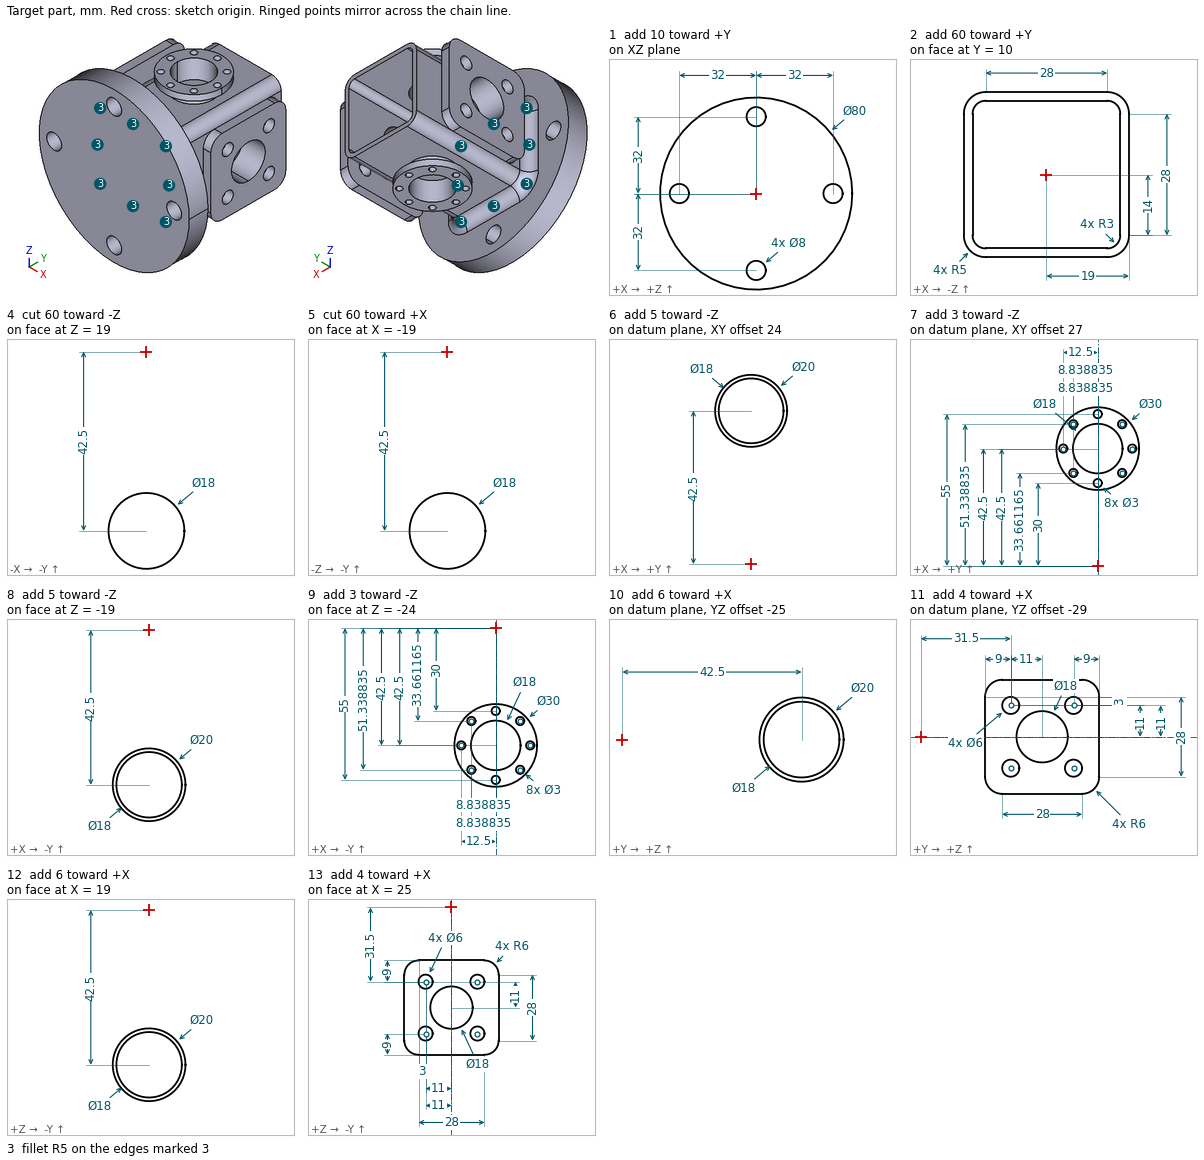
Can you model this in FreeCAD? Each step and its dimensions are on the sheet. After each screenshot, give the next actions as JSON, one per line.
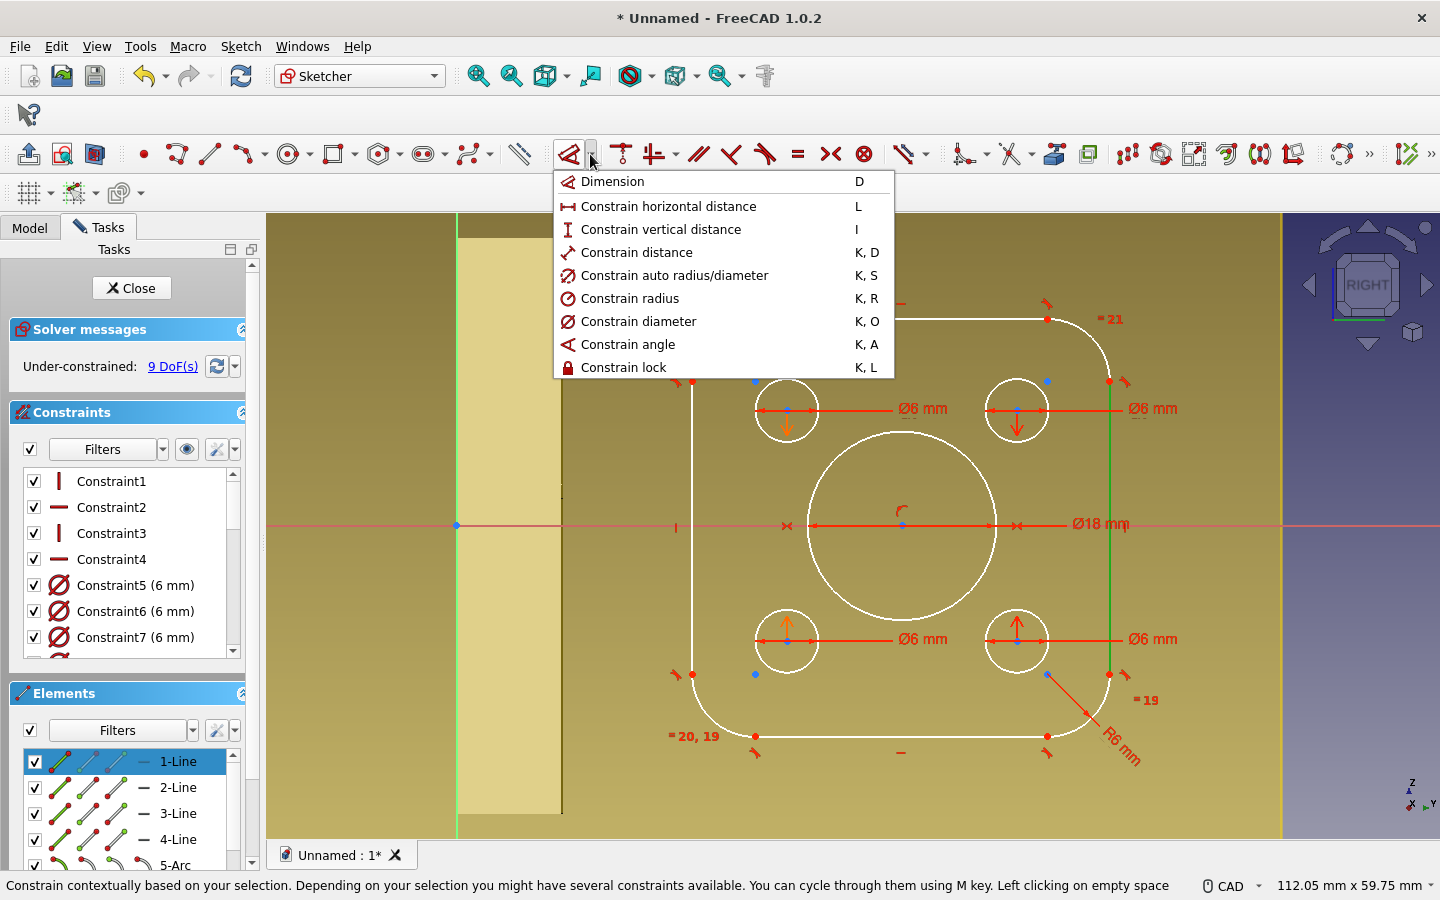
{"action": "left_click", "coordinate": [724, 230]}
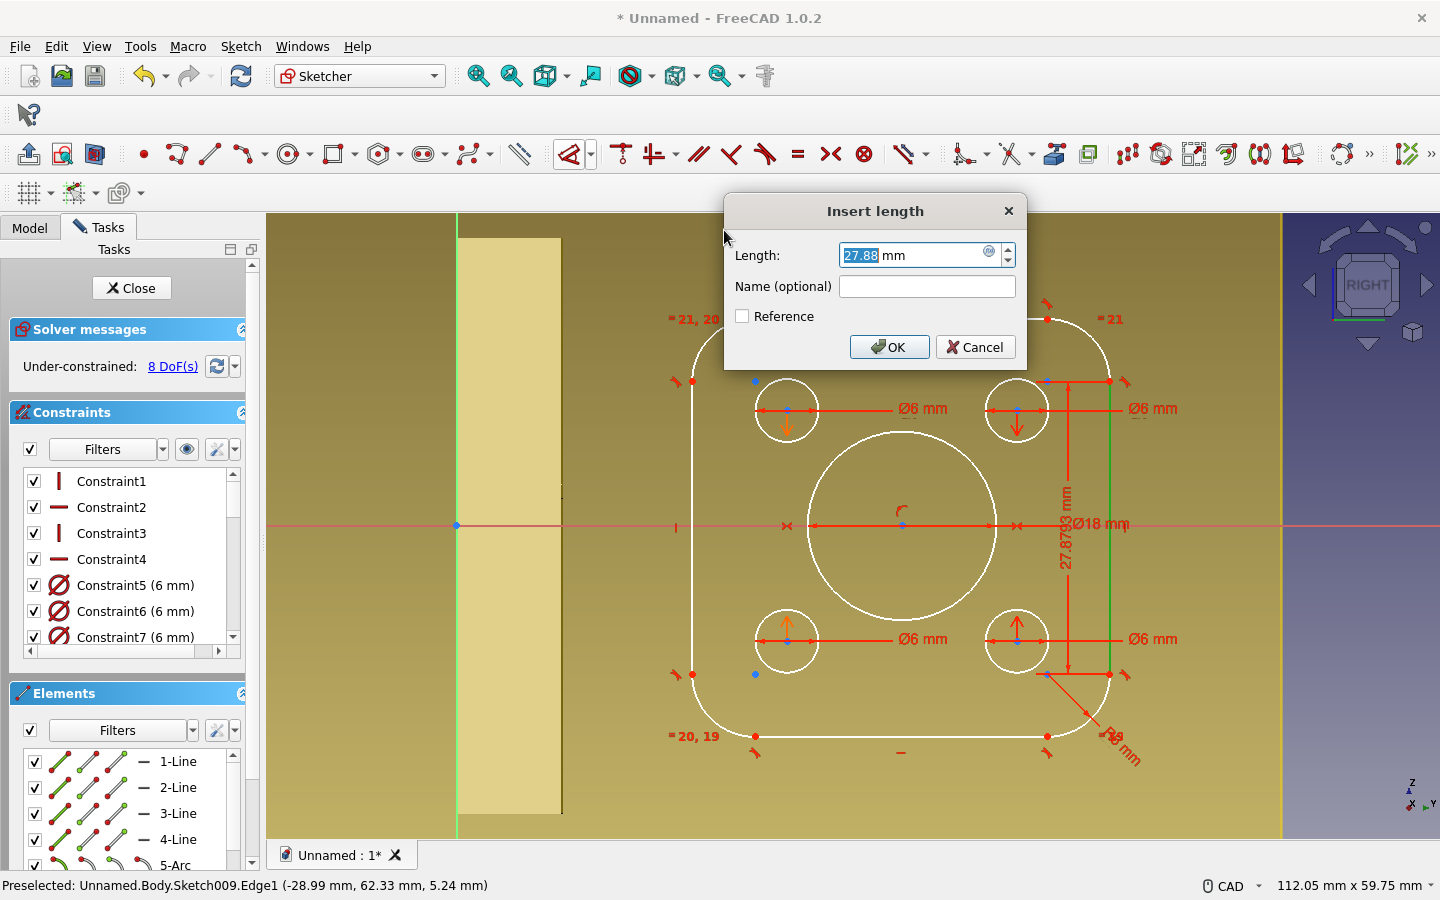
{"action": "type", "text": "28"}
{"action": "key", "text": "Return"}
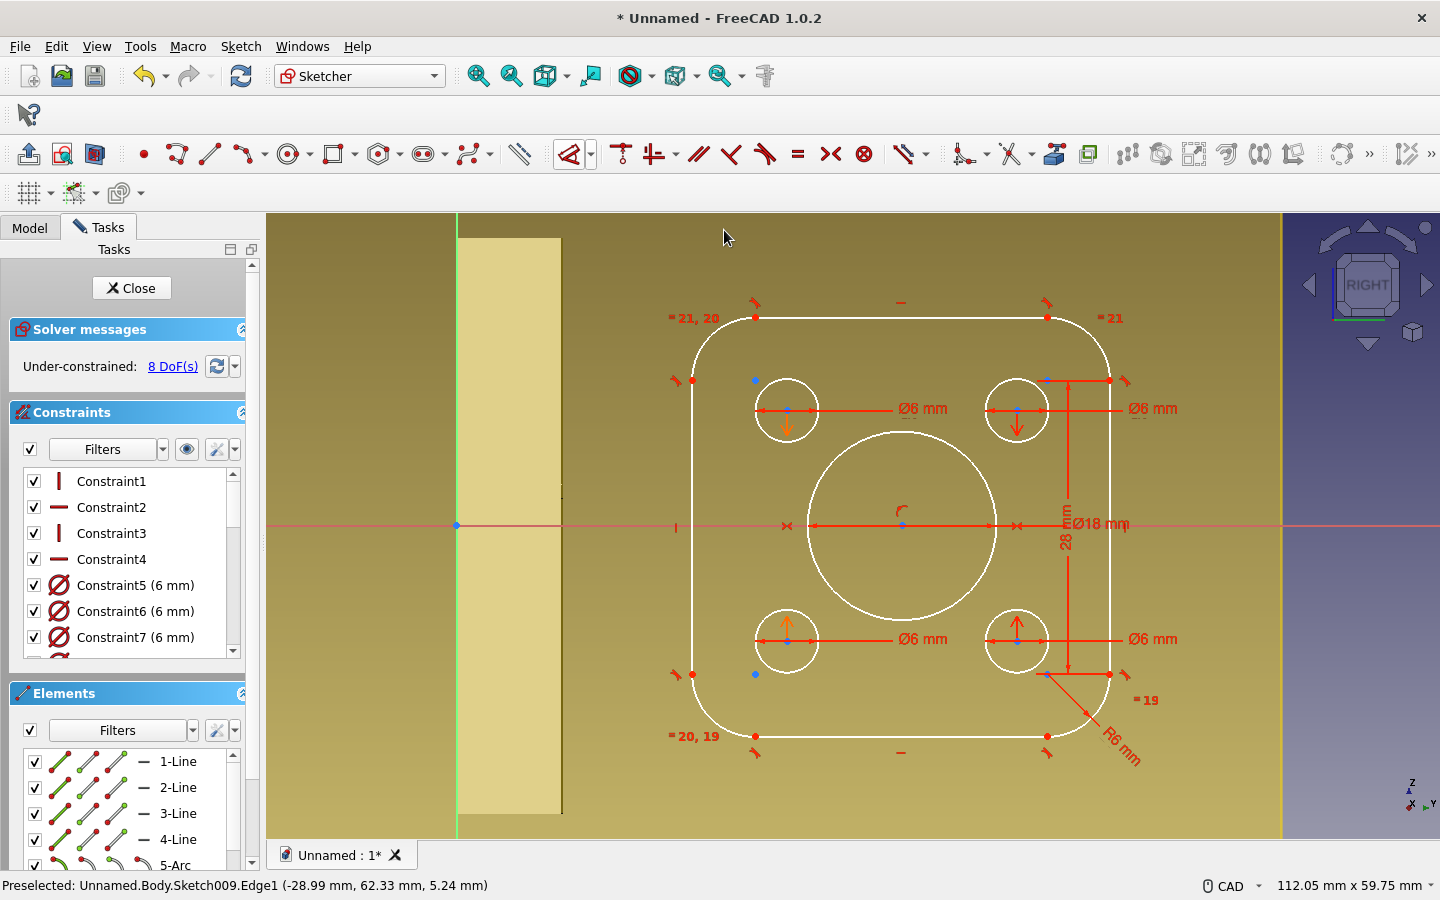
{"action": "left_click", "coordinate": [959, 737]}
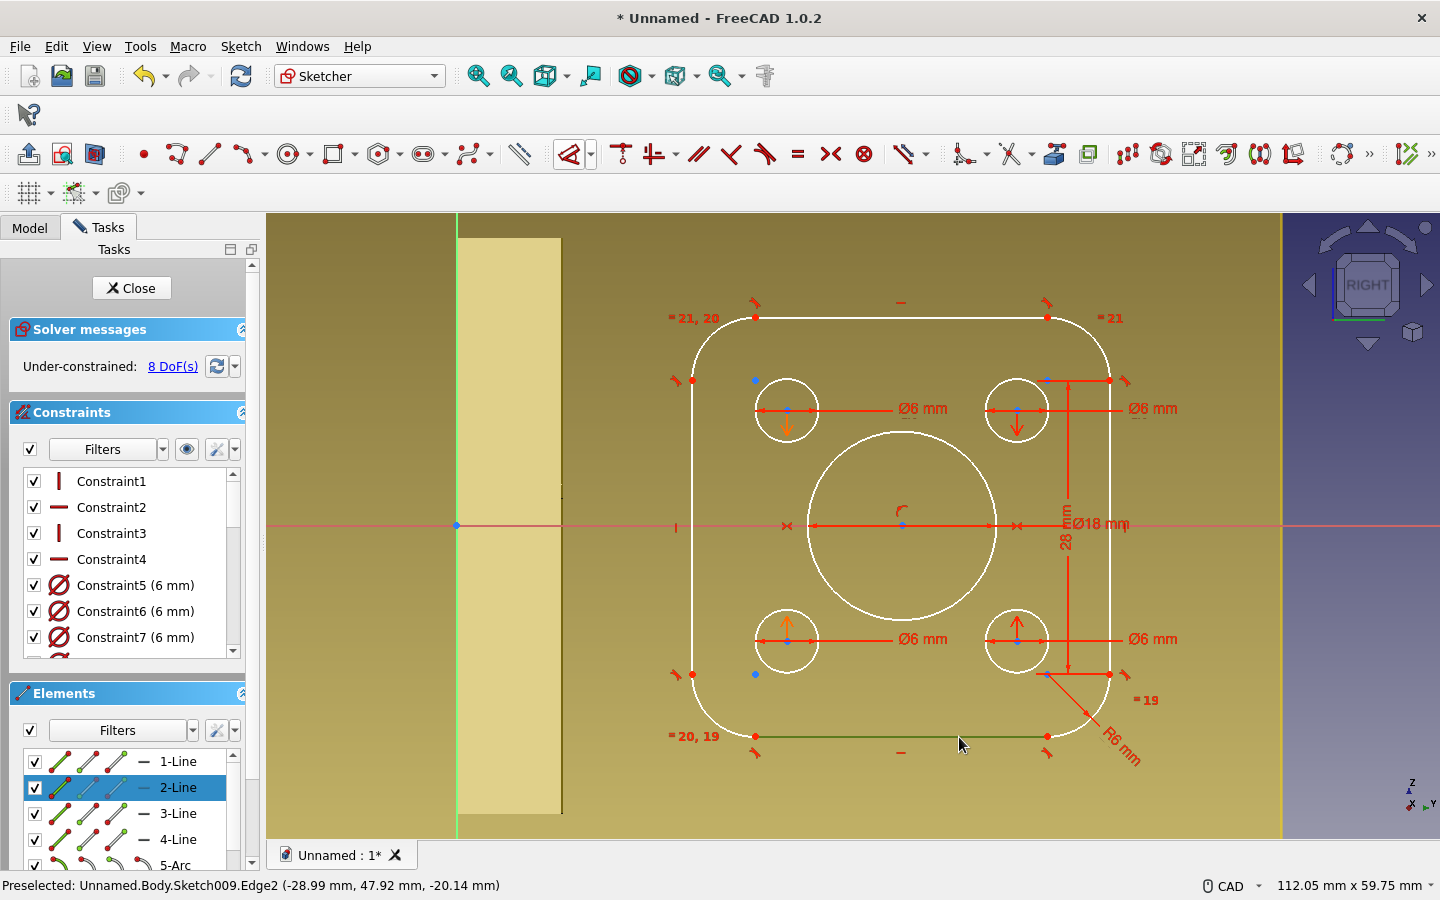
{"action": "left_click", "coordinate": [590, 154]}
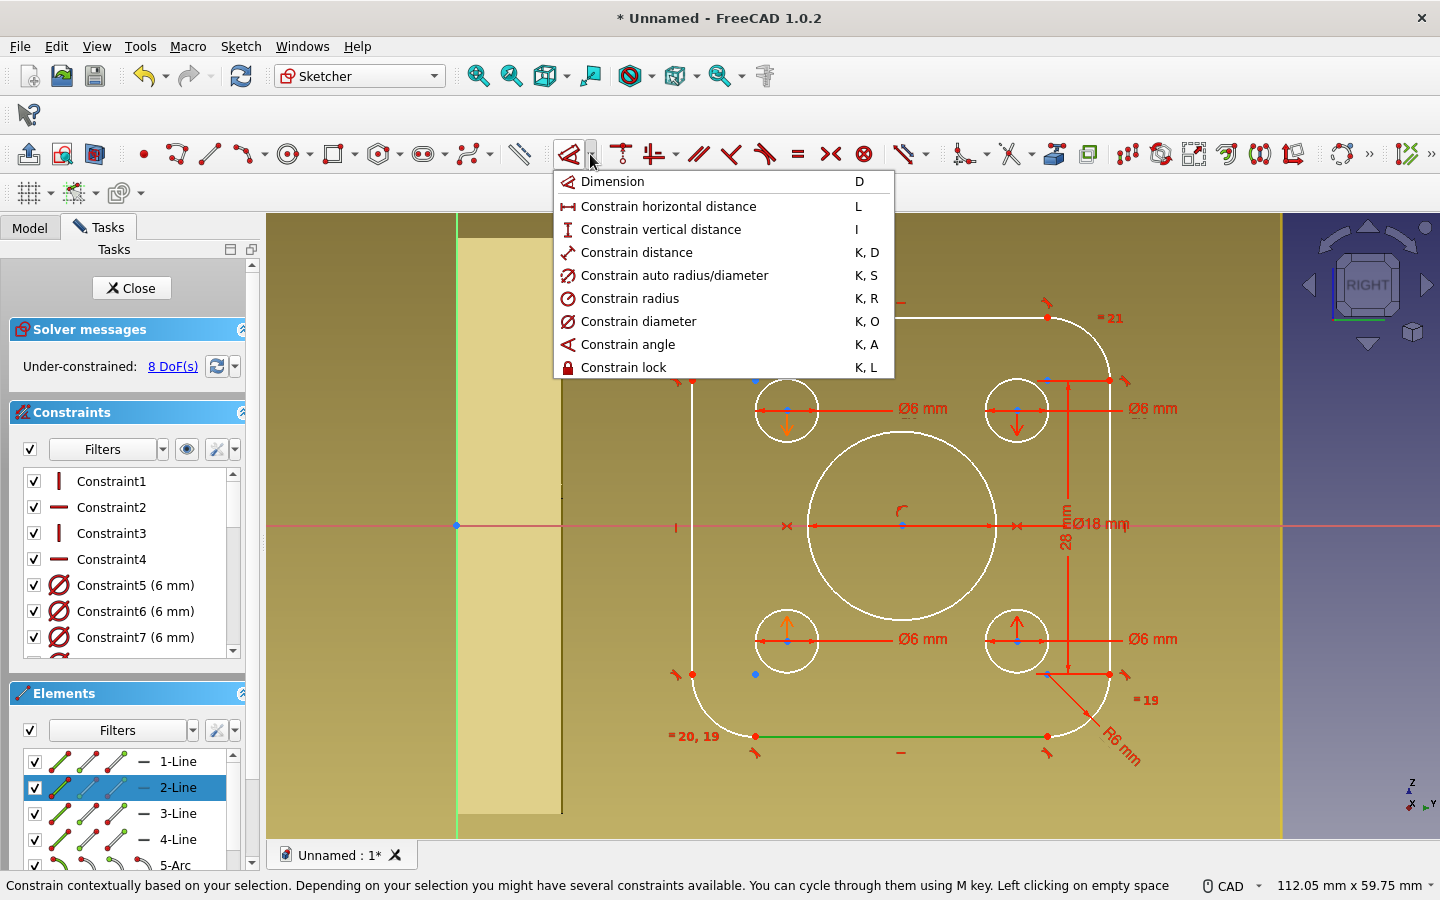
{"action": "left_click", "coordinate": [724, 206]}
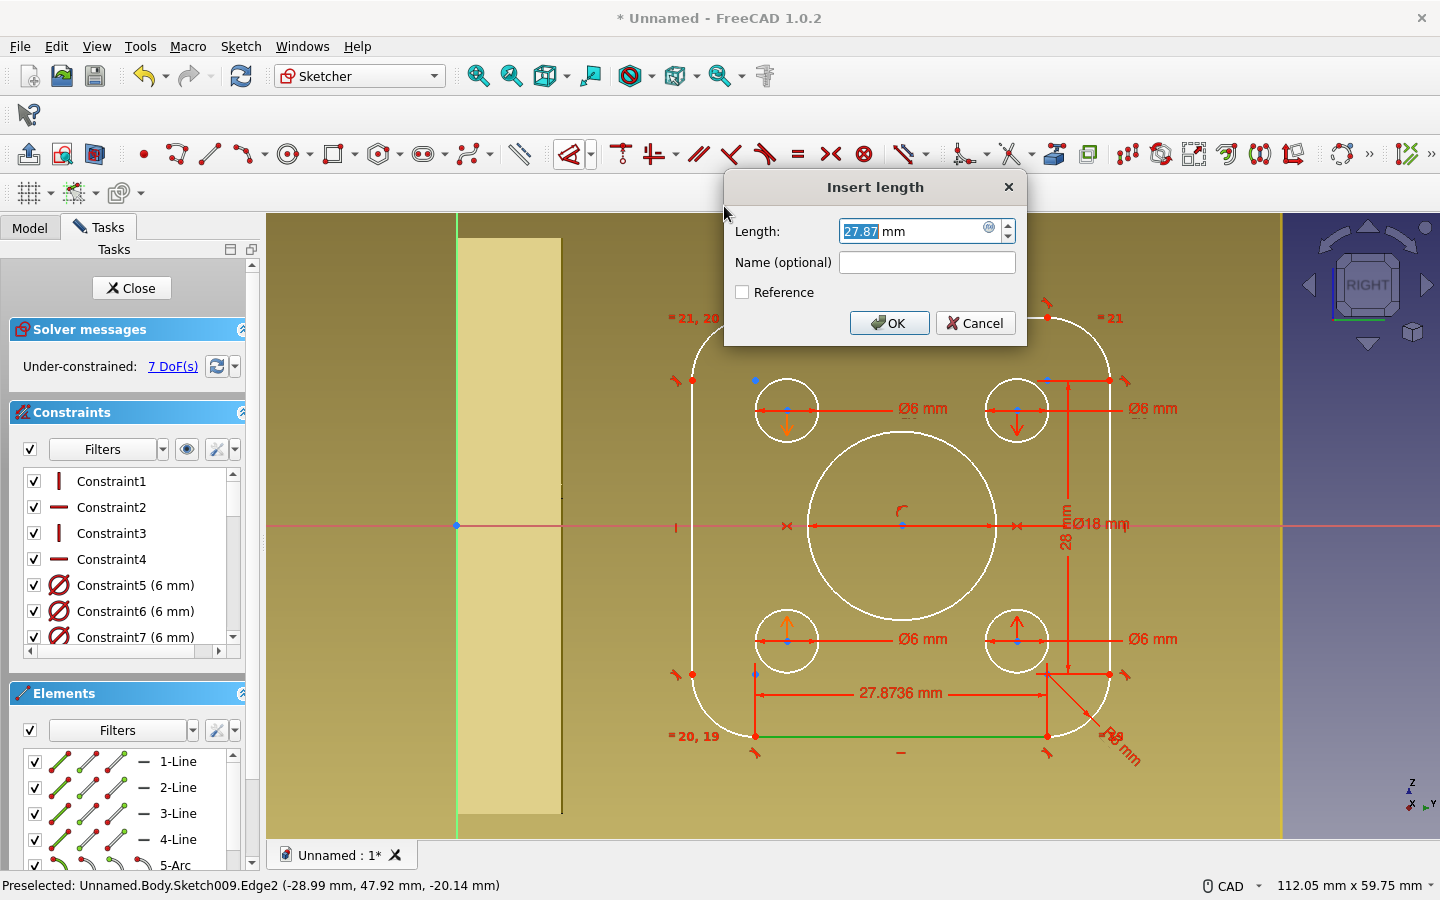
{"action": "type", "text": "28"}
{"action": "key", "text": "Return"}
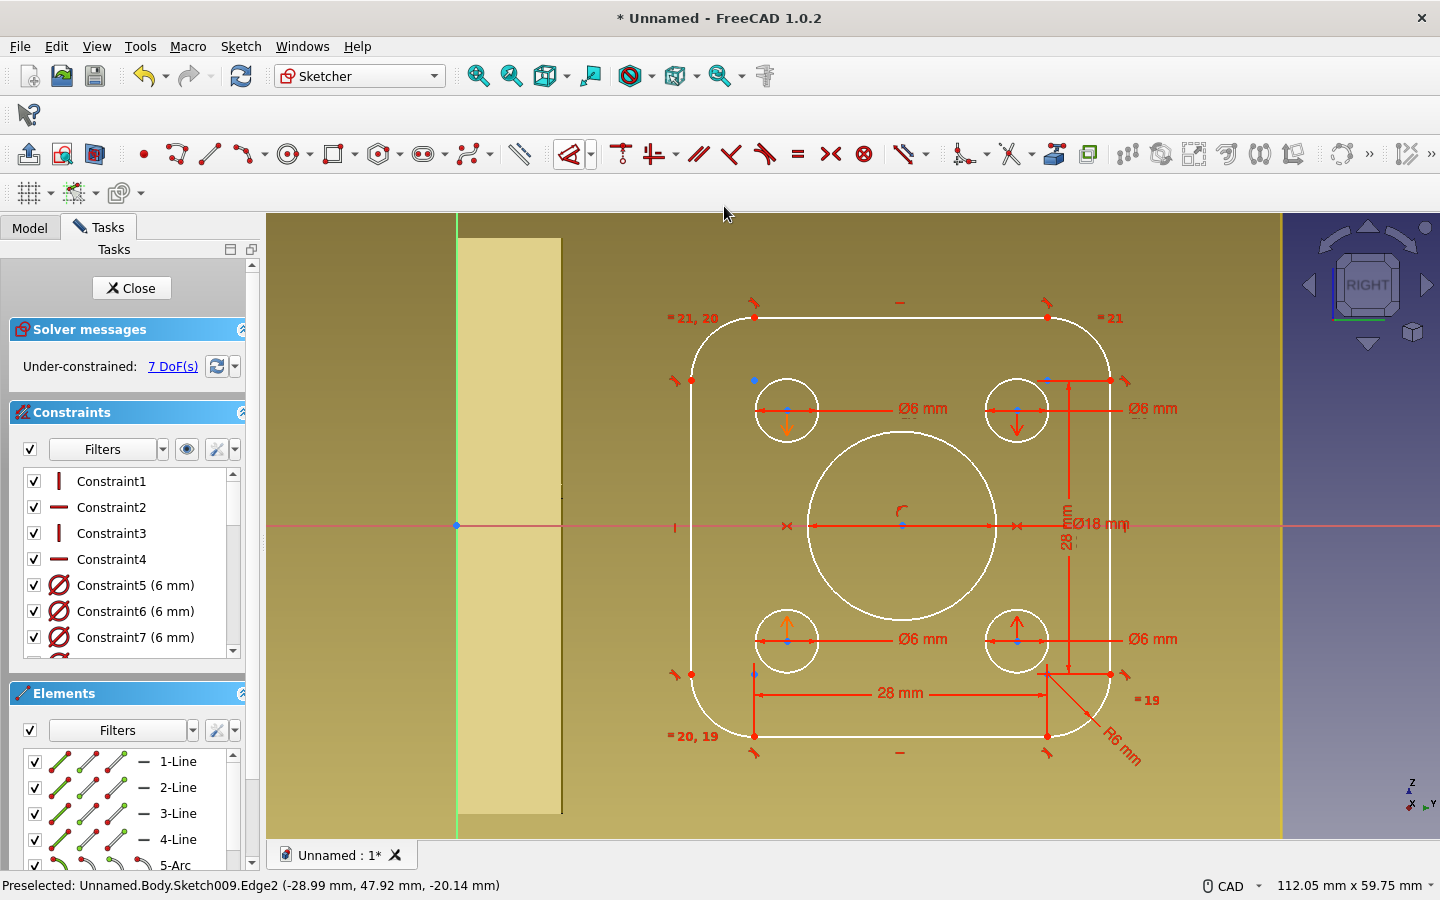
{"action": "left_click", "coordinate": [787, 411]}